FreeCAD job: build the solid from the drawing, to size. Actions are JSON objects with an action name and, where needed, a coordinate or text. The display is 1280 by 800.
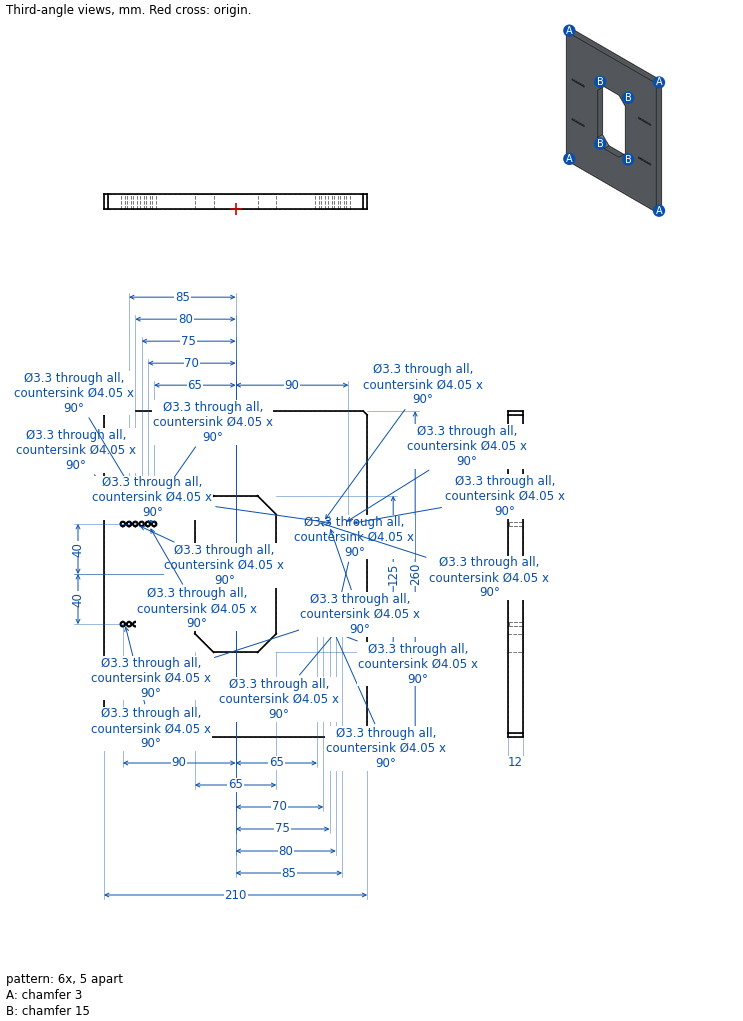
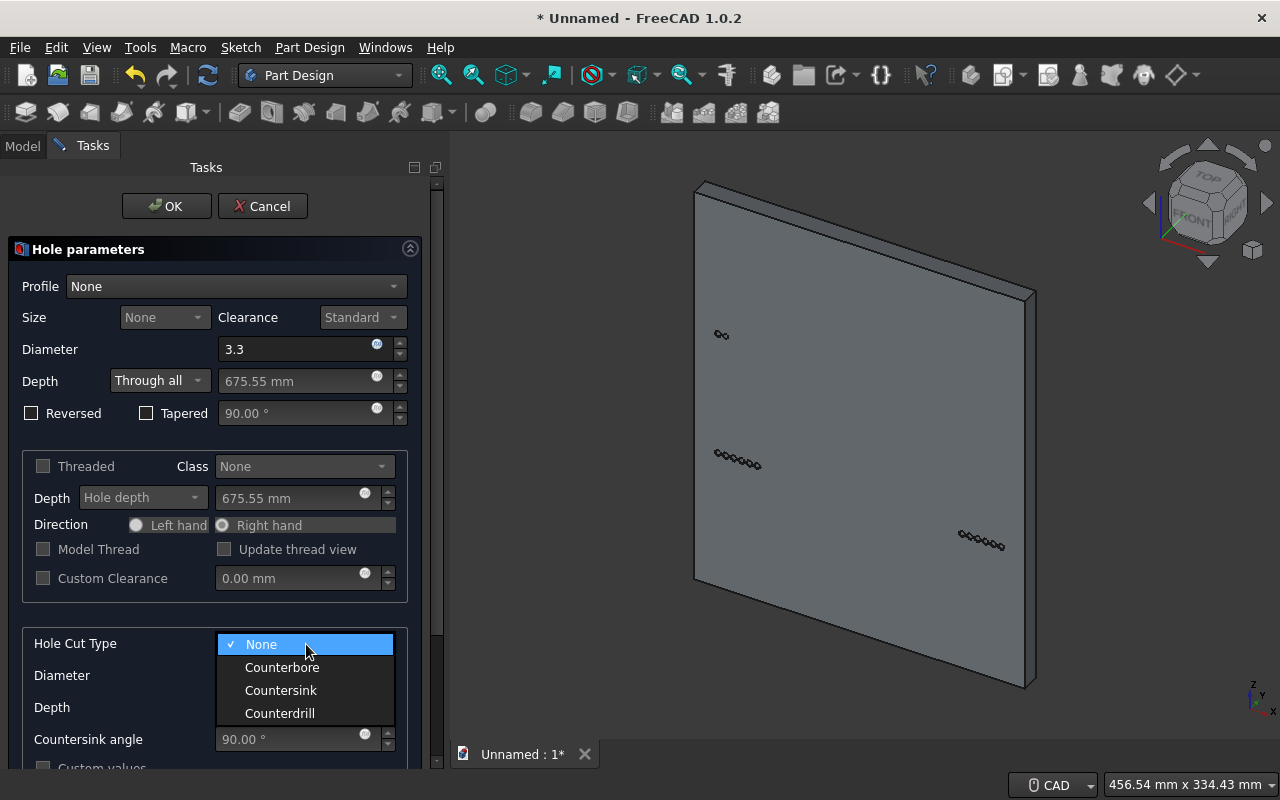
{"action": "left_click", "coordinate": [304, 690]}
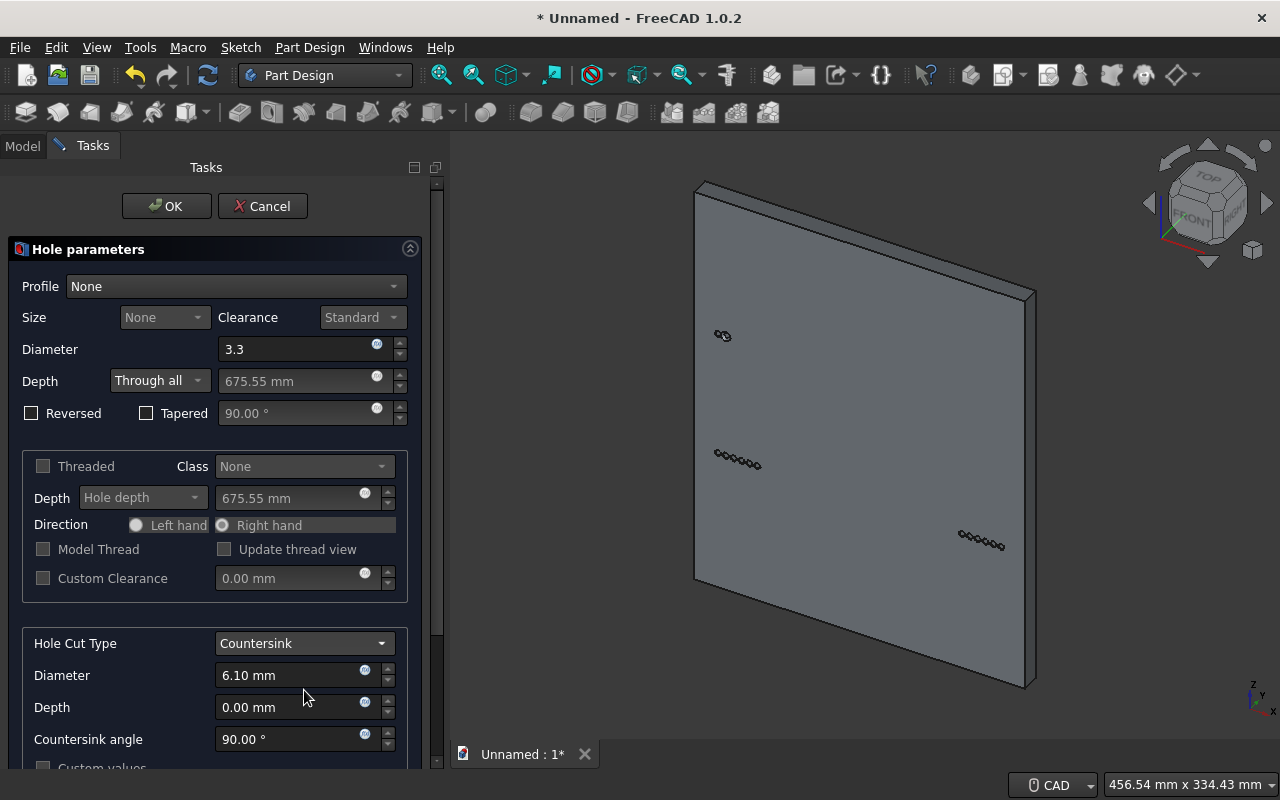
{"action": "triple_click", "coordinate": [298, 675]}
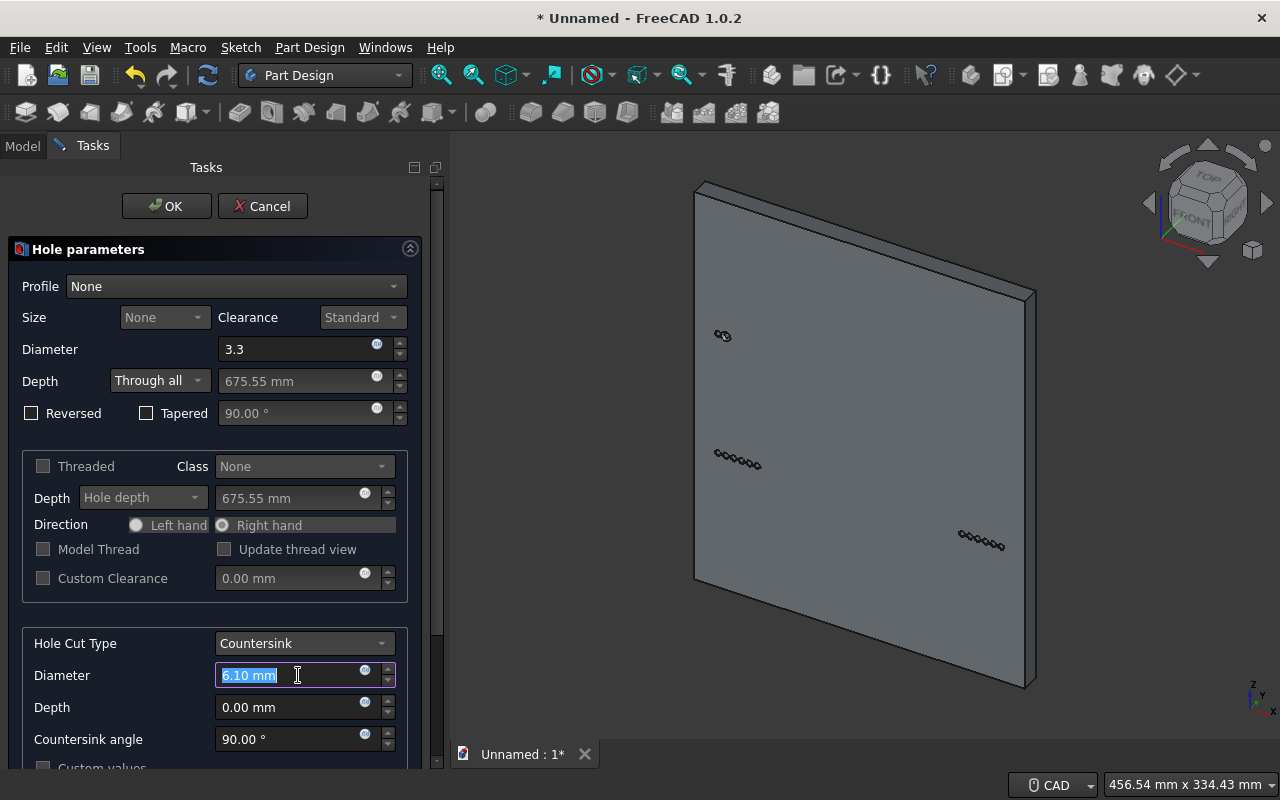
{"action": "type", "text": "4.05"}
{"action": "key", "text": "Tab"}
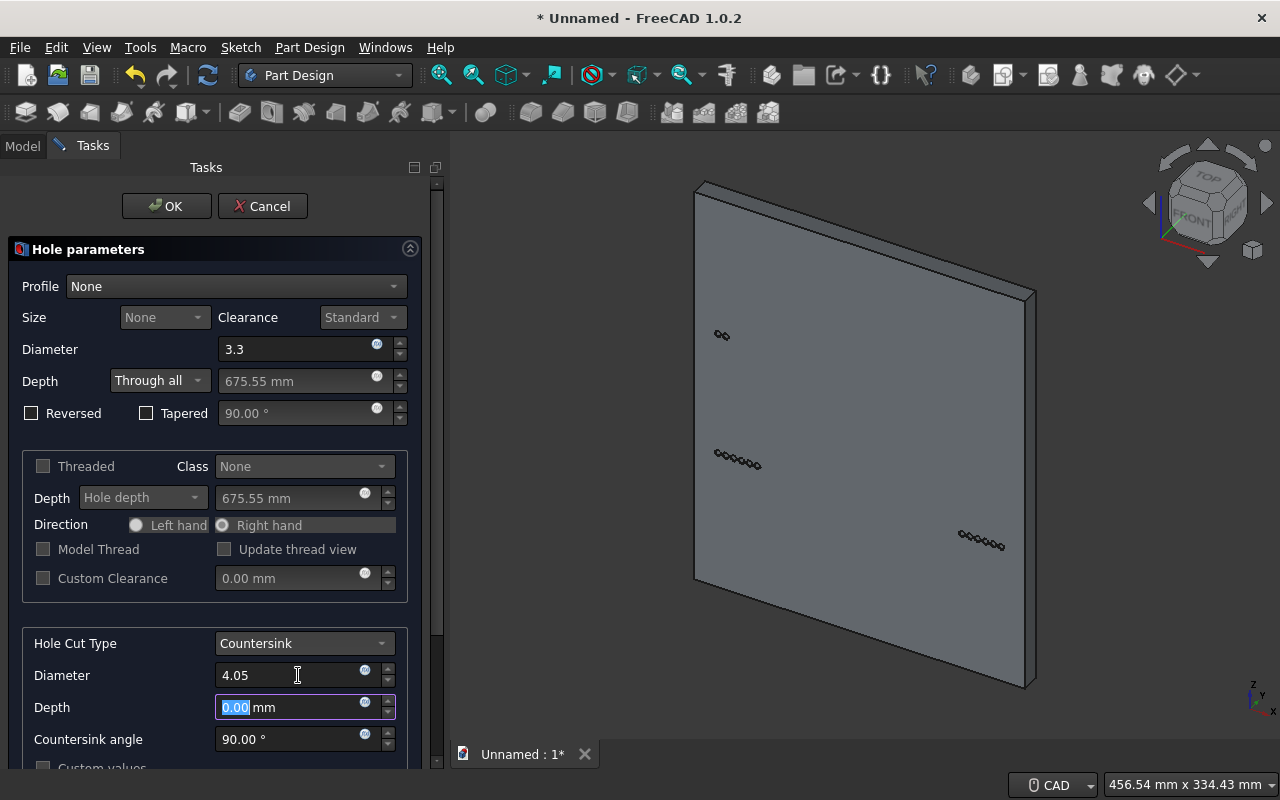
{"action": "left_click", "coordinate": [167, 206]}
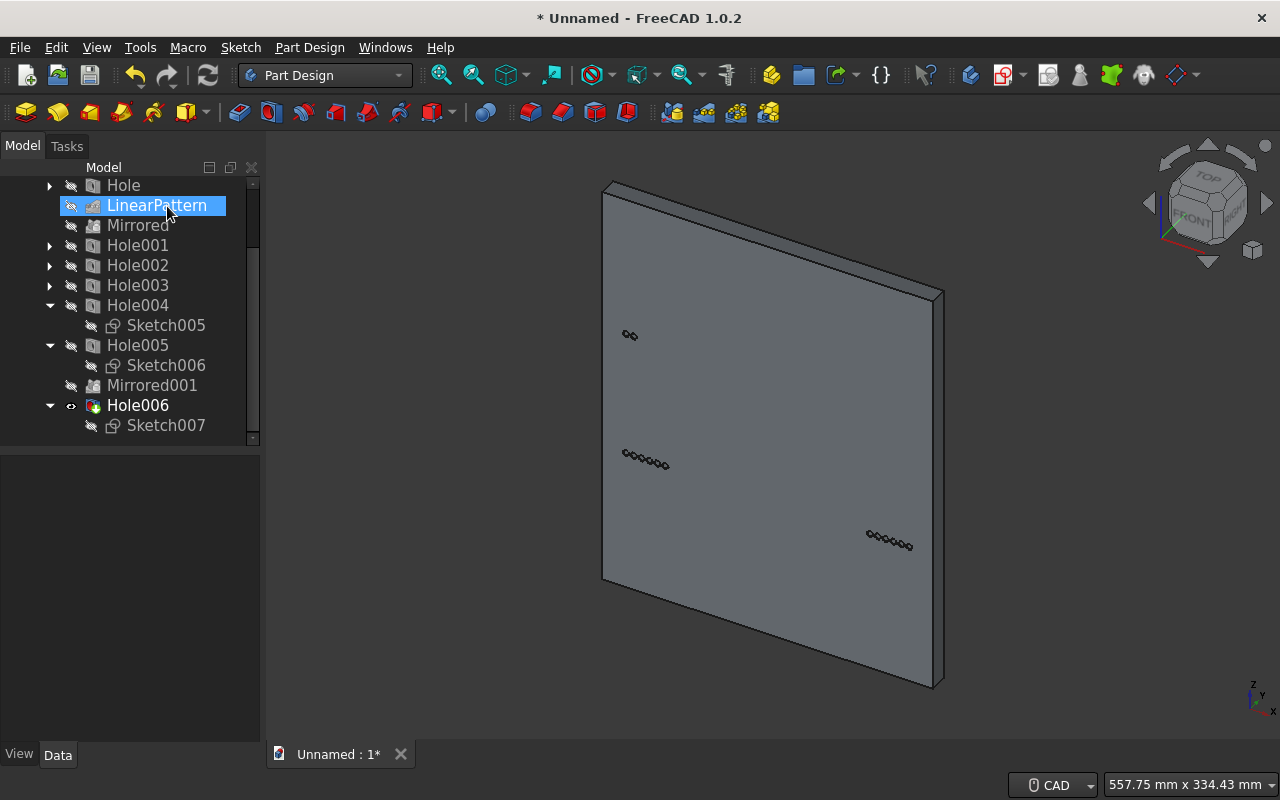
{"action": "left_click", "coordinate": [1004, 76]}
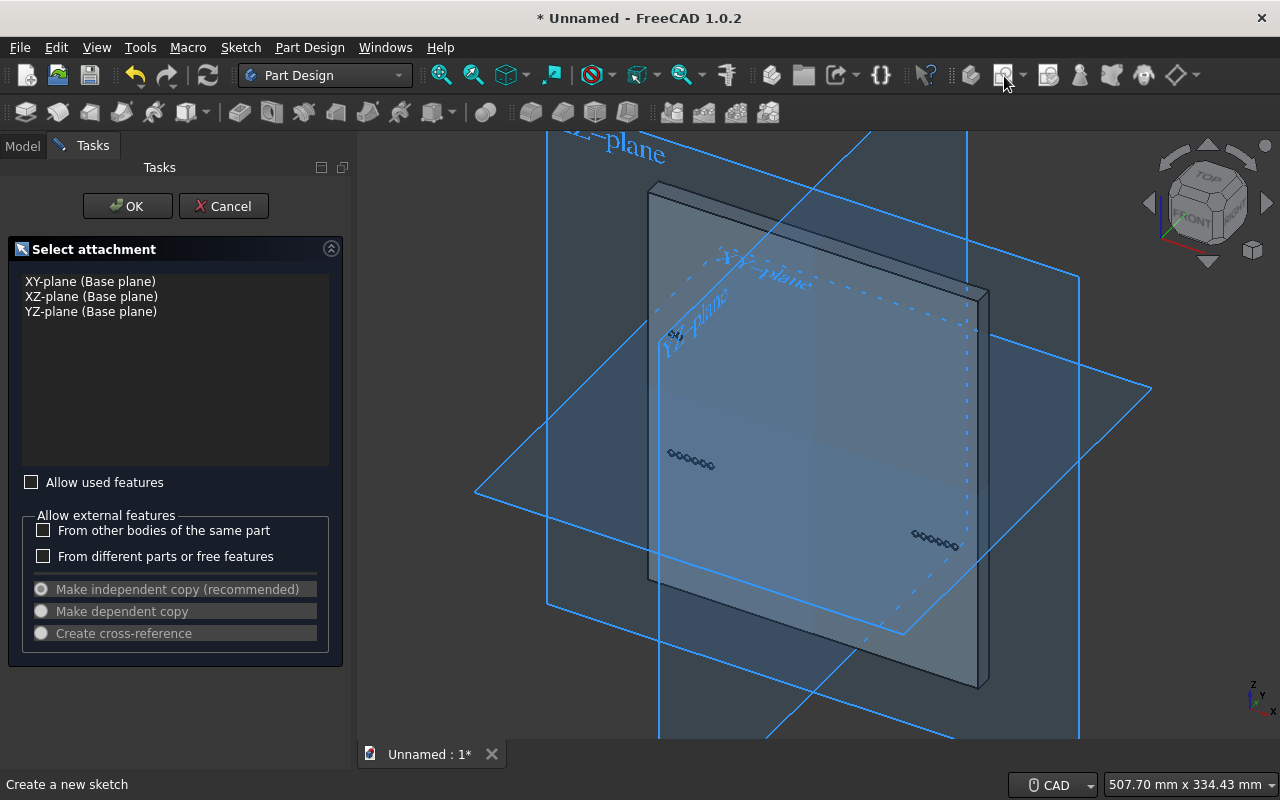
{"action": "left_click", "coordinate": [82, 296]}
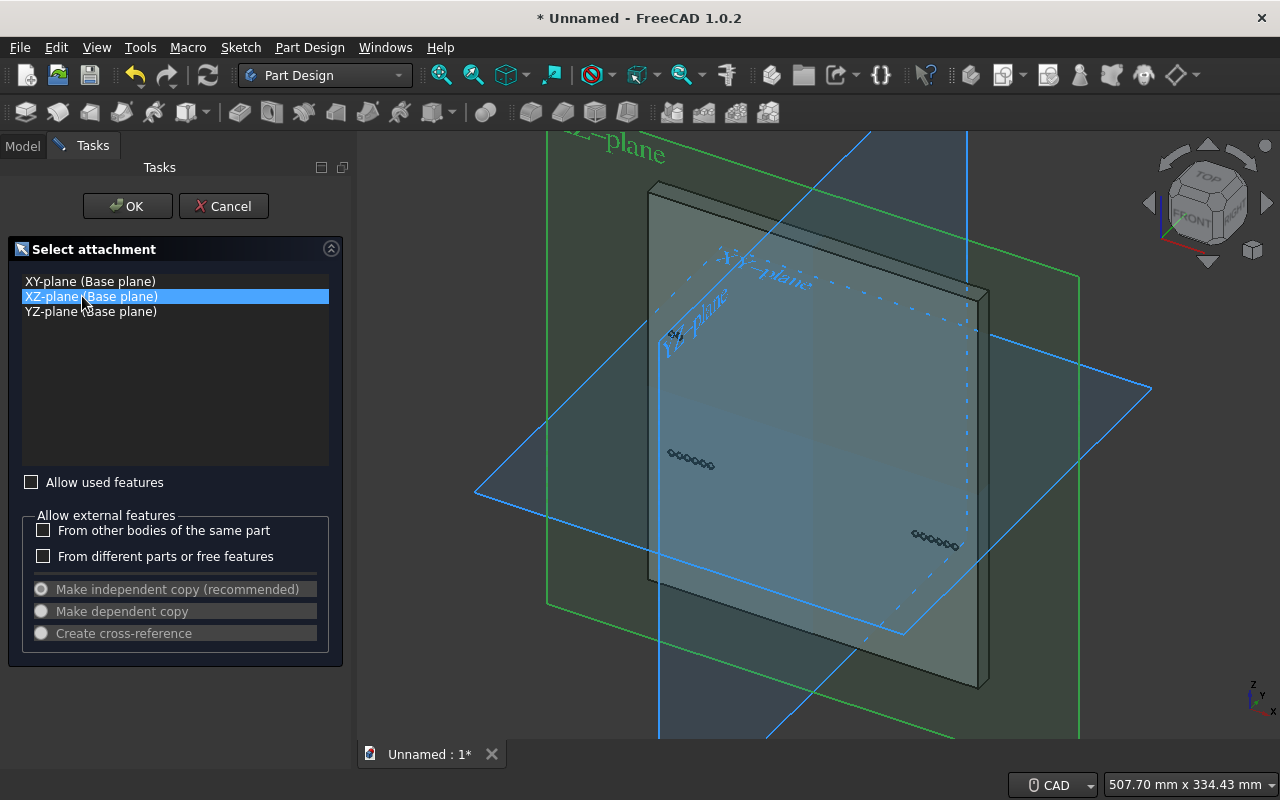
{"action": "left_click", "coordinate": [128, 206]}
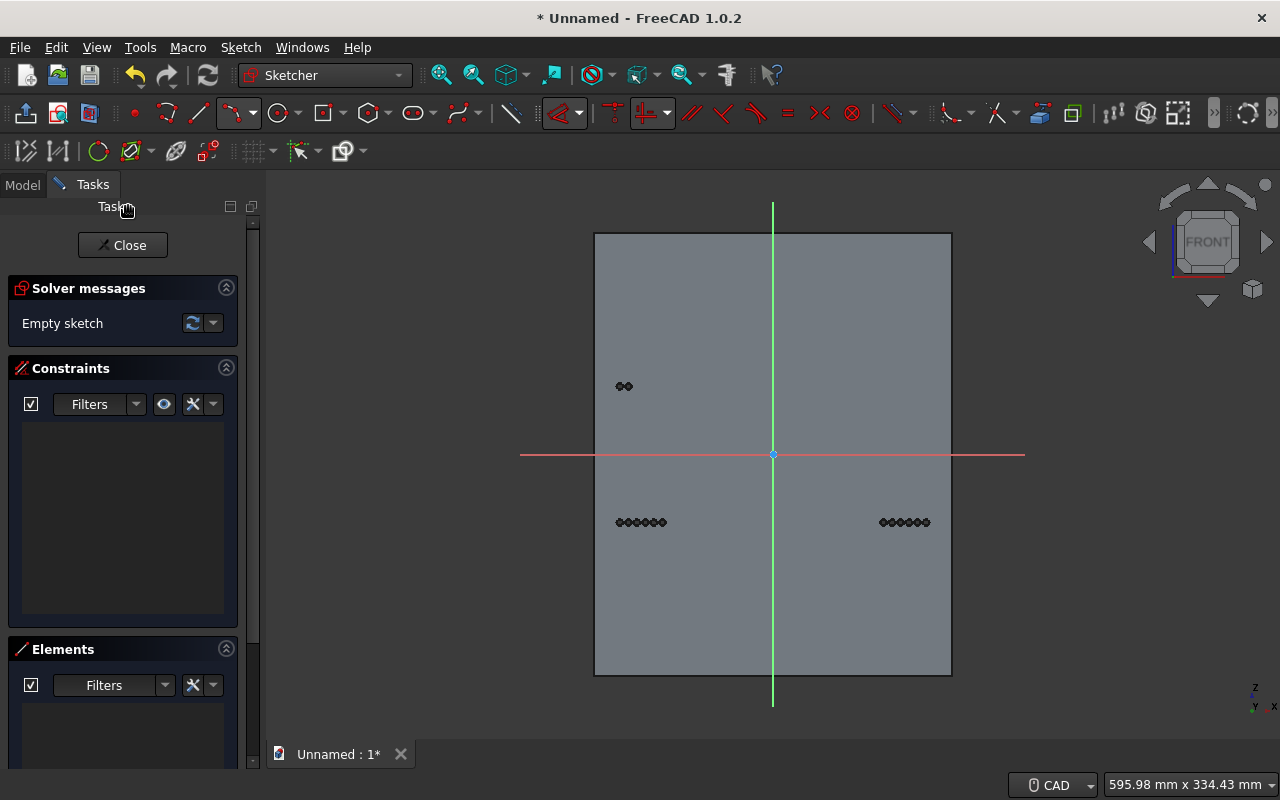
{"action": "scroll", "coordinate": [633, 383], "scroll_direction": "up", "scroll_amount": 15}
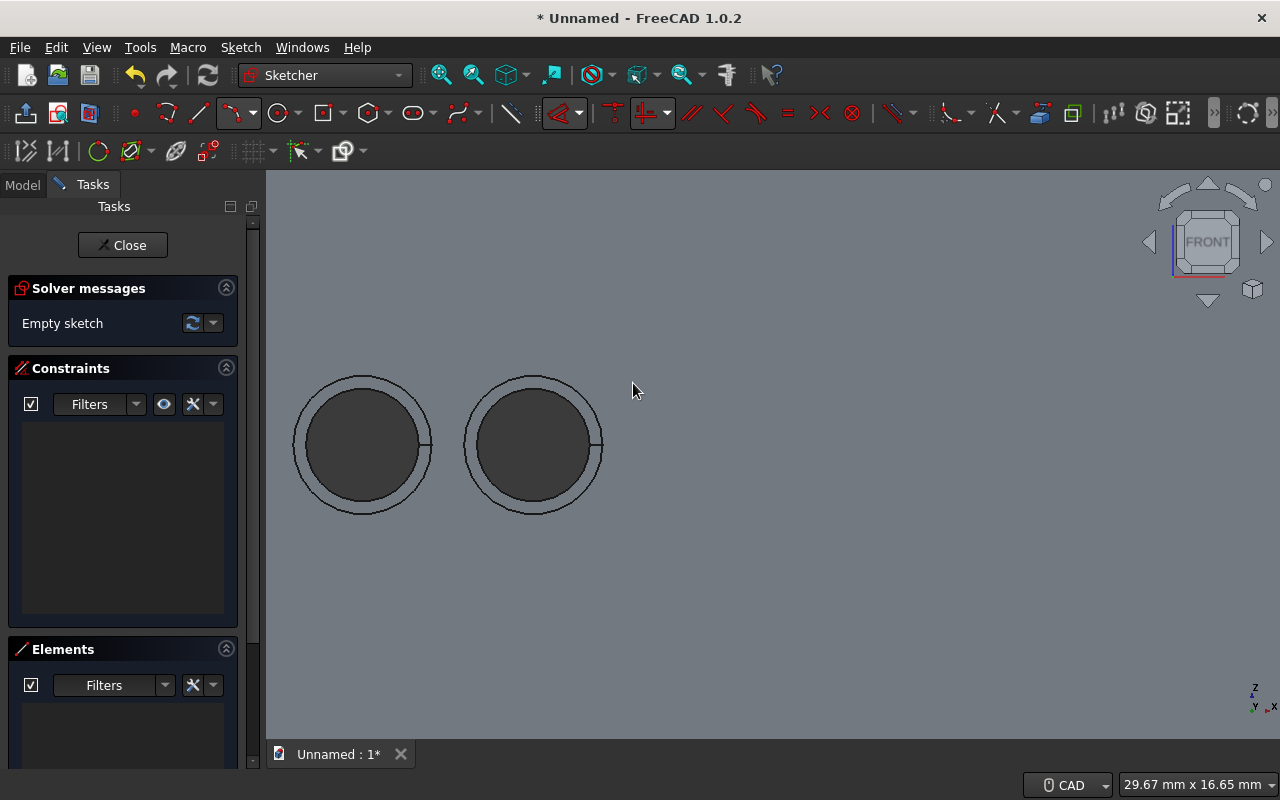
{"action": "scroll", "coordinate": [704, 441], "scroll_direction": "up", "scroll_amount": 6}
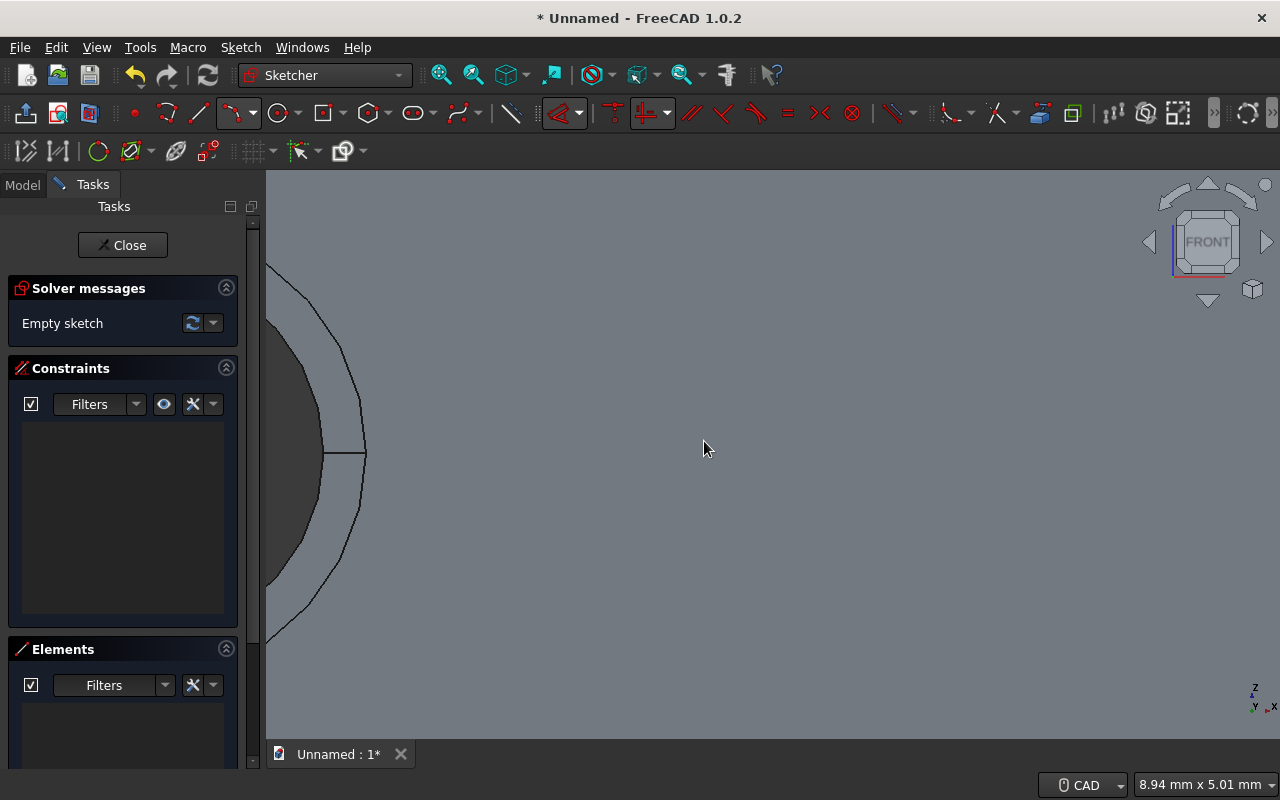
{"action": "left_click", "coordinate": [278, 114]}